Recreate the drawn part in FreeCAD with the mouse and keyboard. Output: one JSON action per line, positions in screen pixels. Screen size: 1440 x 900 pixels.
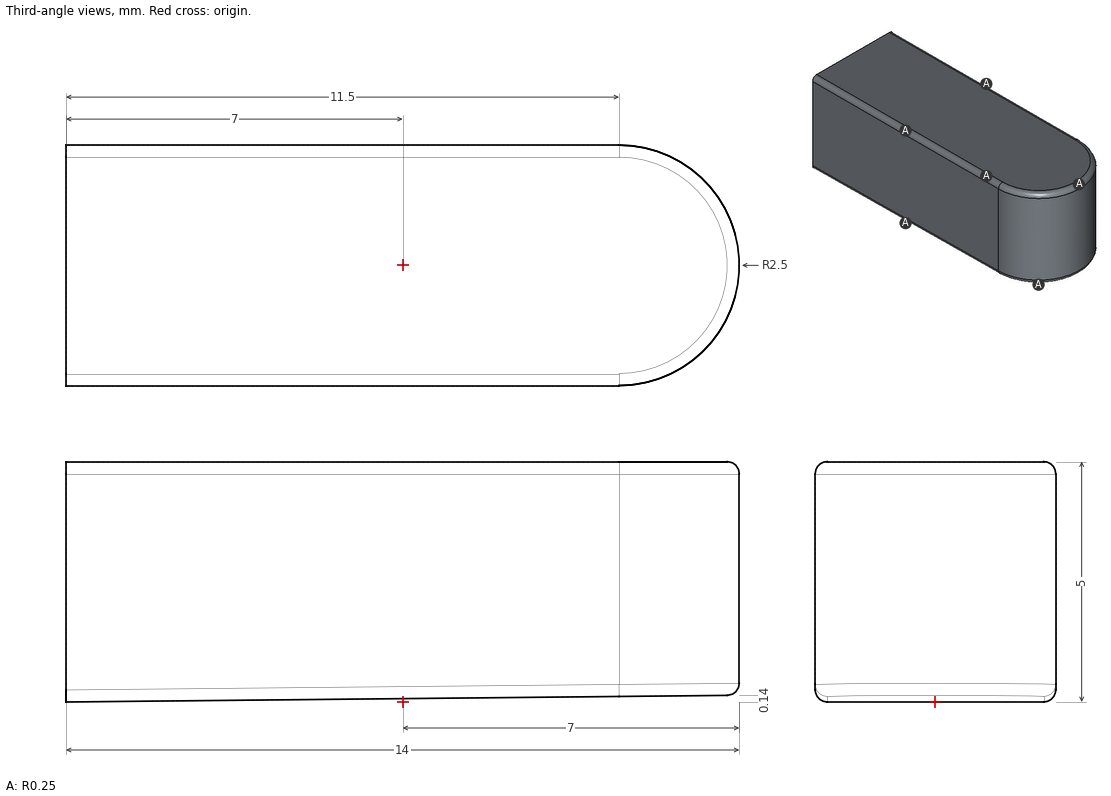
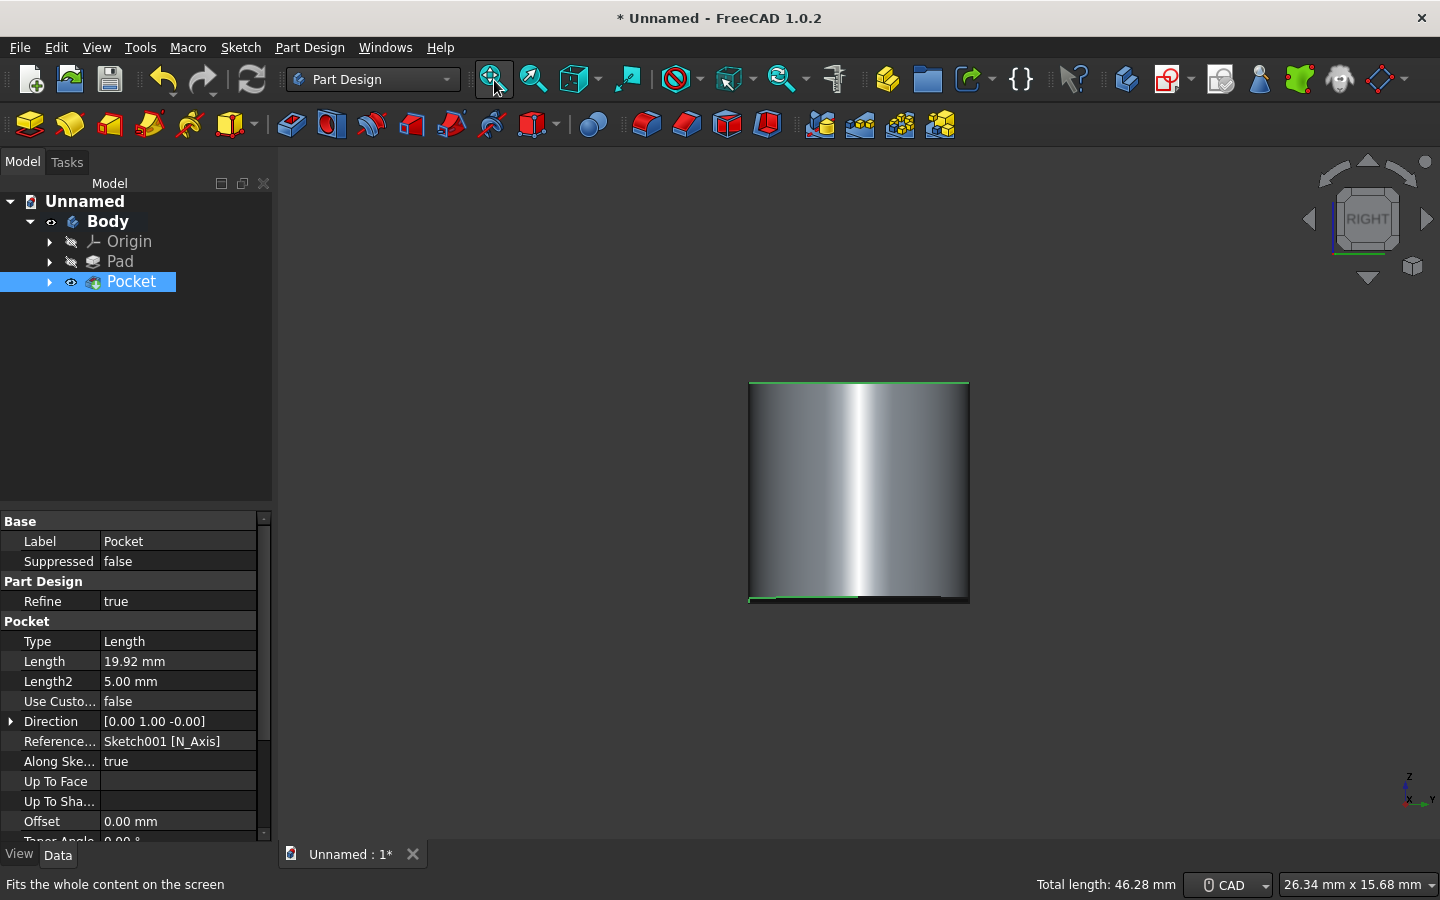
{"action": "key", "text": "5"}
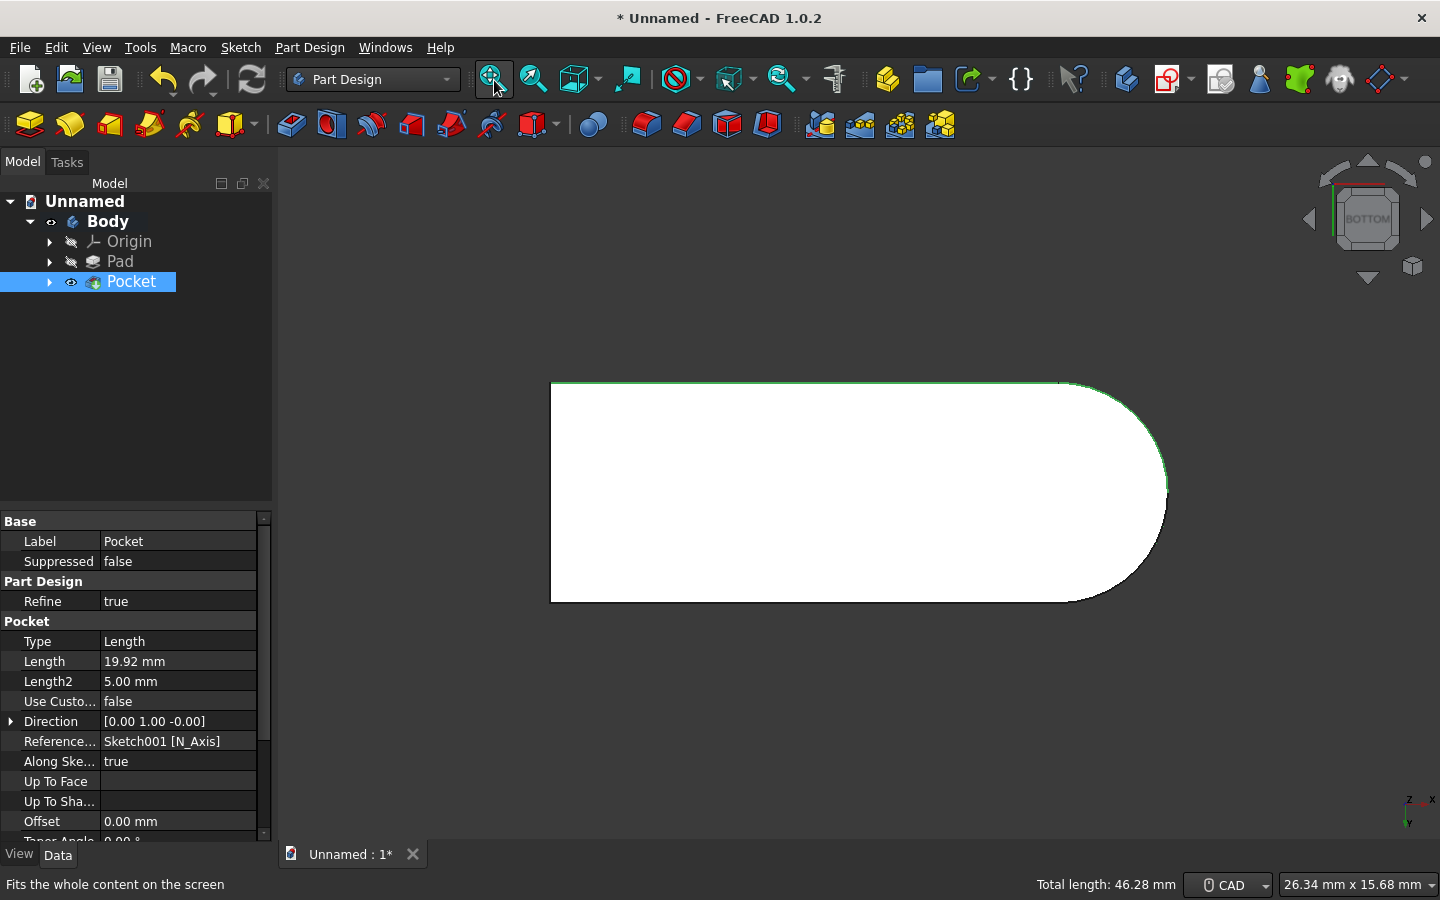
{"action": "left_click", "coordinate": [804, 602], "text": "ctrl"}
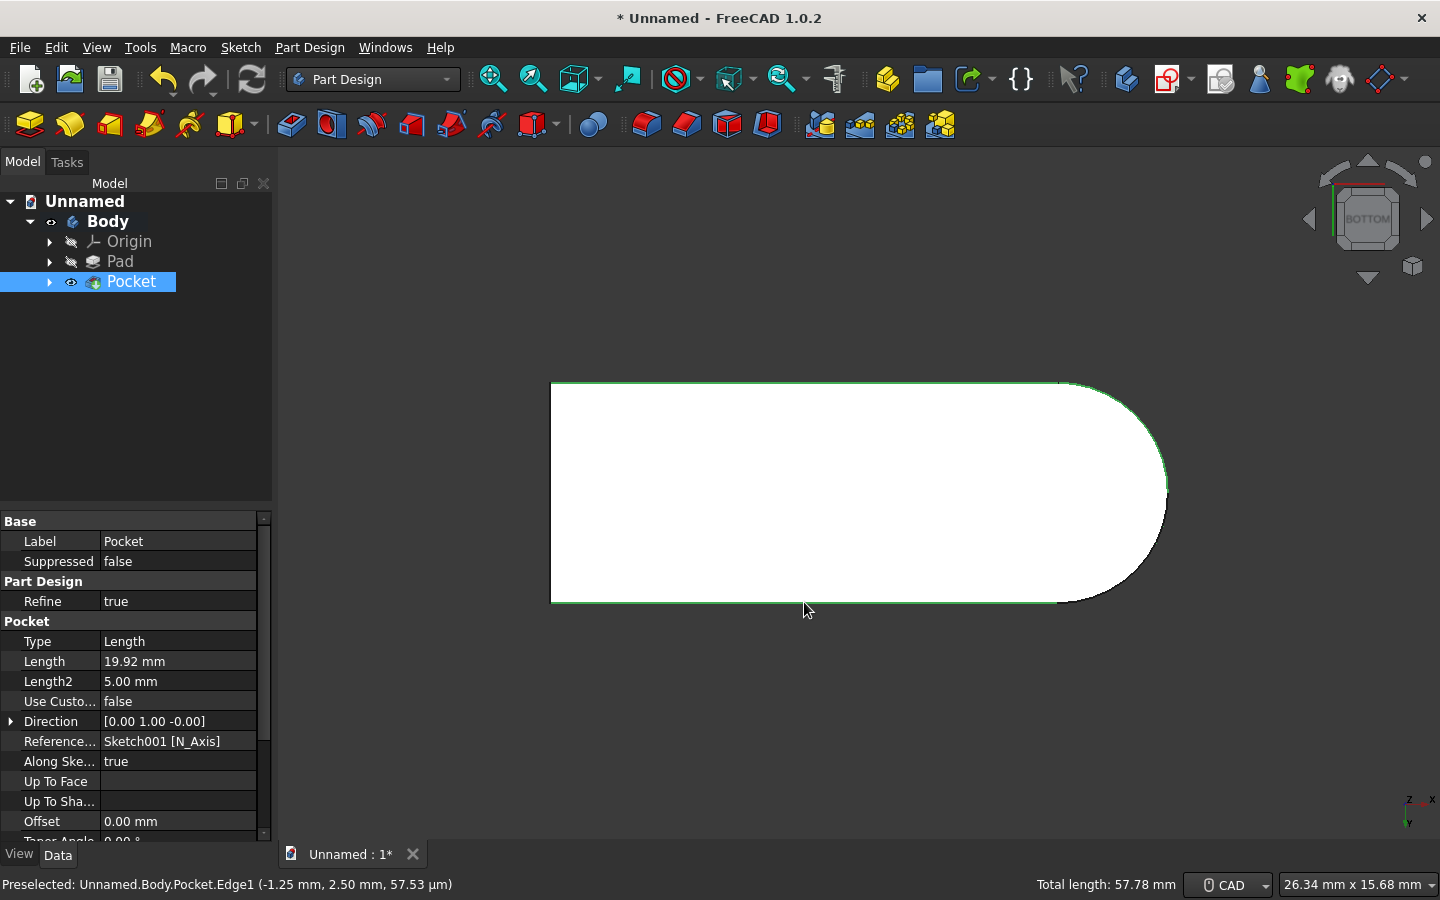
{"action": "left_click", "coordinate": [648, 124]}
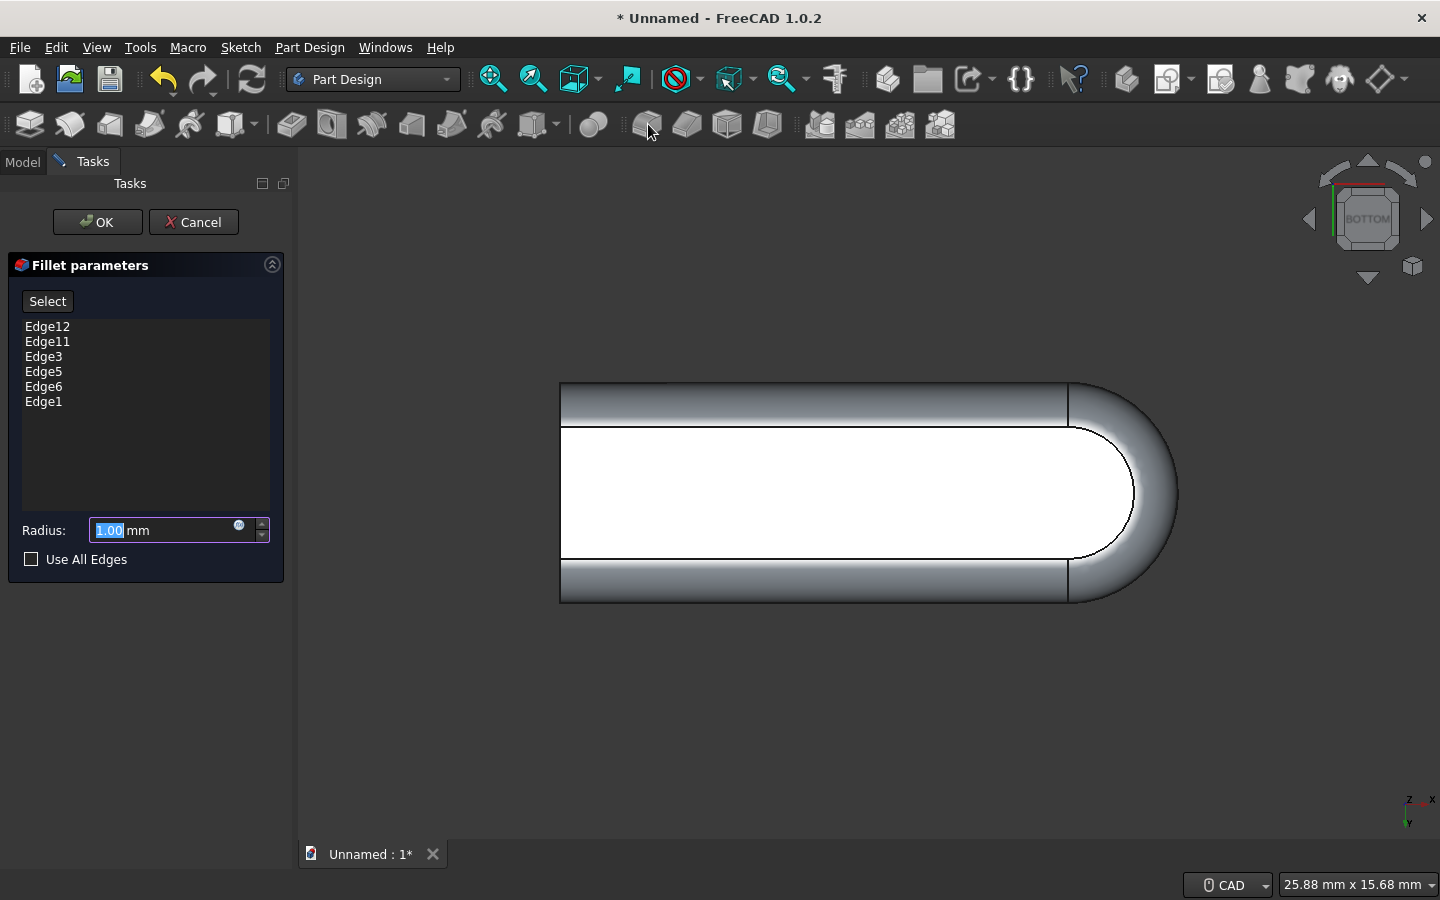
{"action": "type", "text": "0.25"}
{"action": "key", "text": "Tab"}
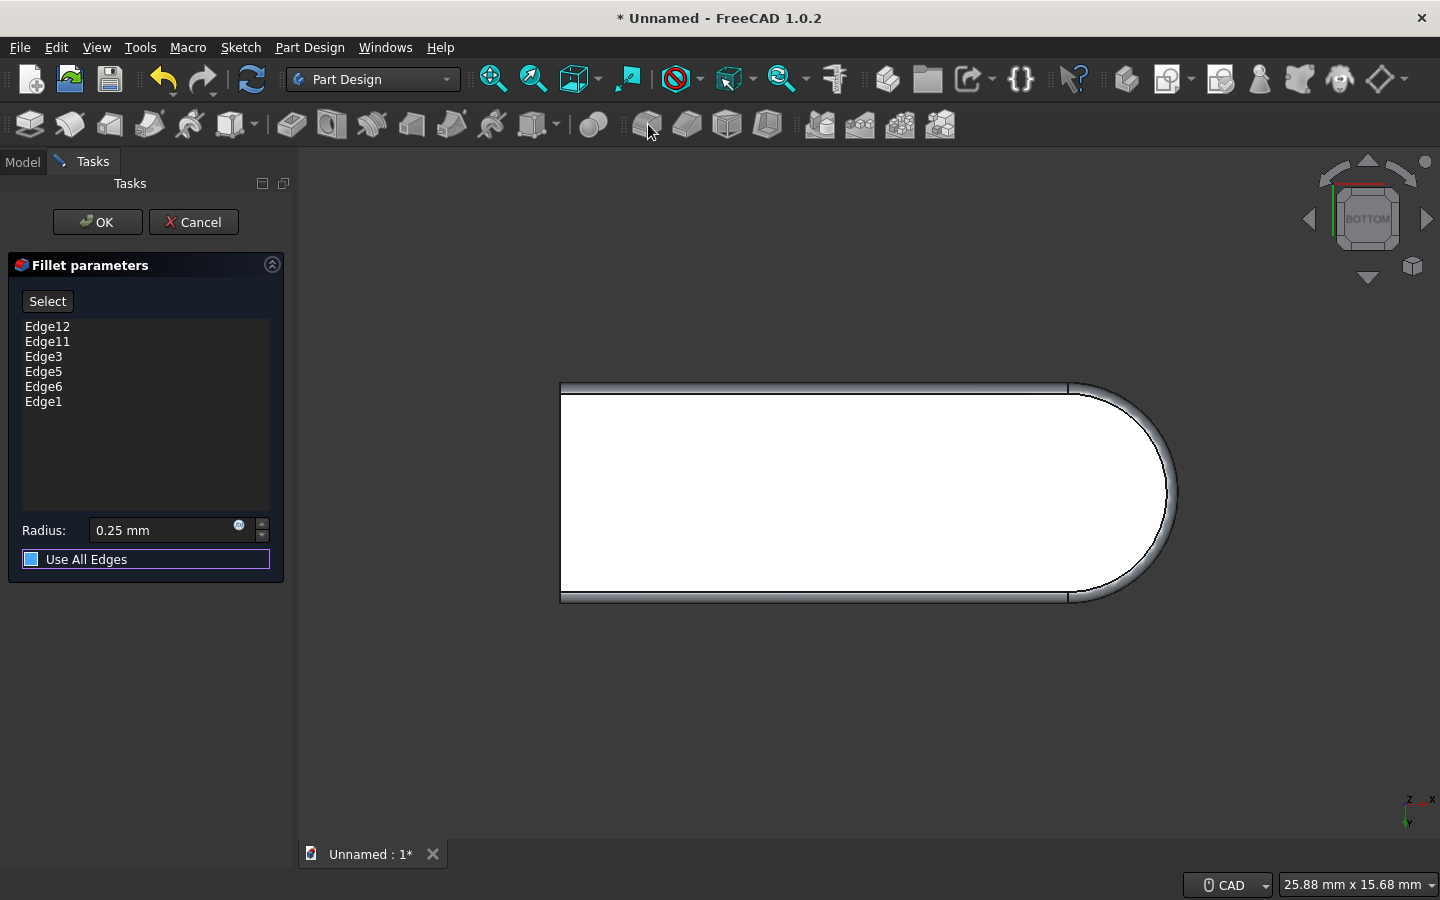
{"action": "left_click", "coordinate": [98, 222]}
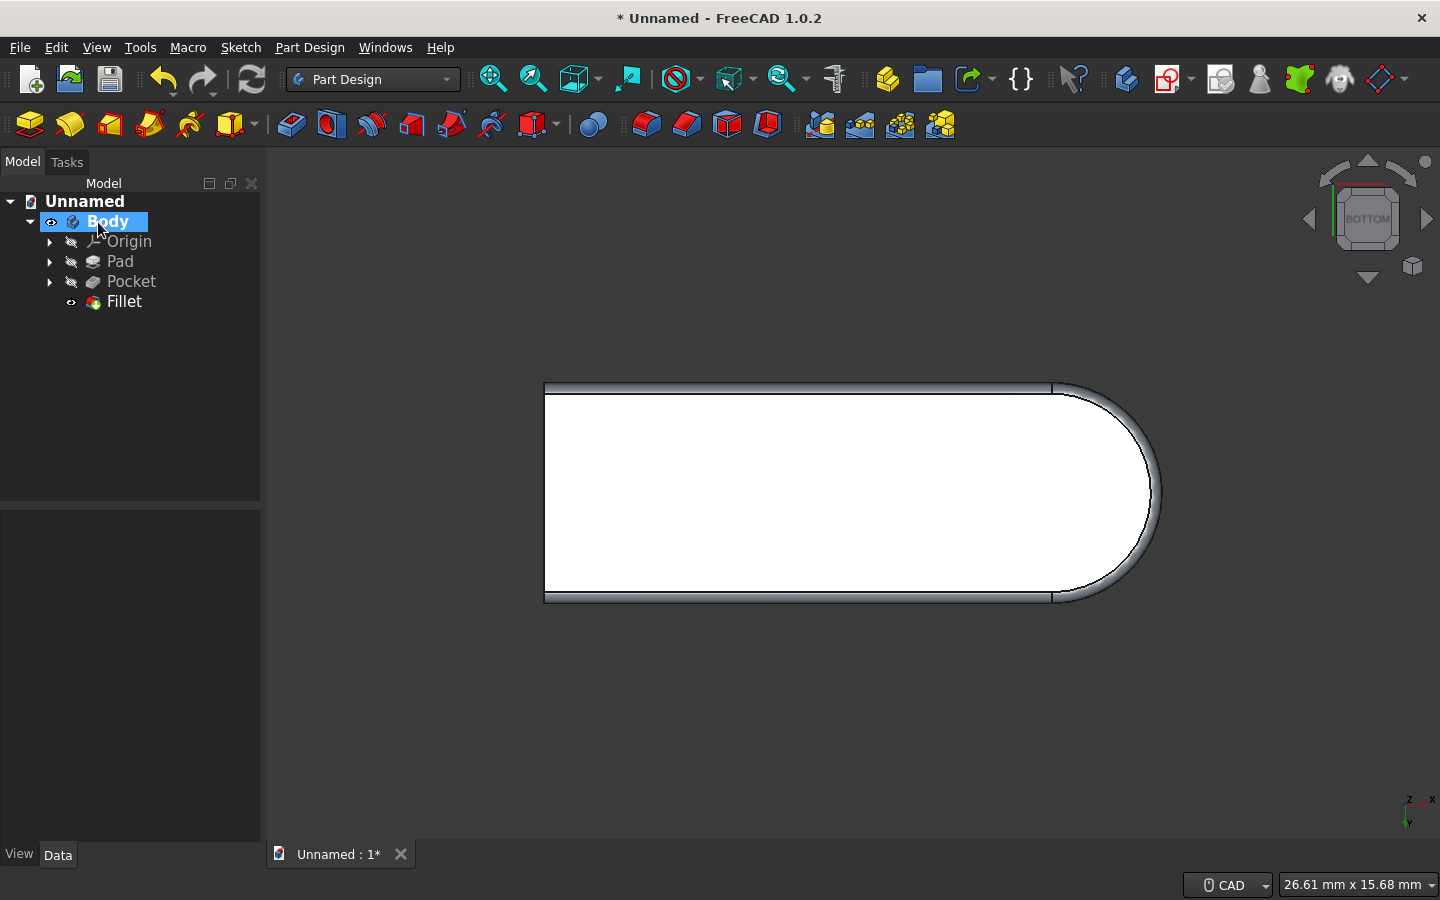
{"action": "key", "text": "0"}